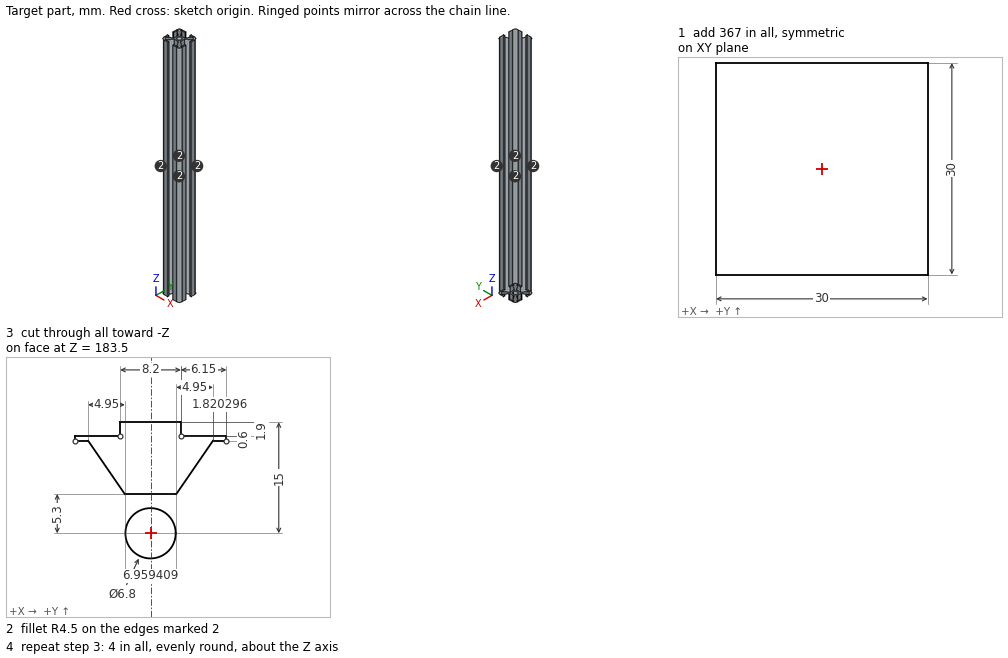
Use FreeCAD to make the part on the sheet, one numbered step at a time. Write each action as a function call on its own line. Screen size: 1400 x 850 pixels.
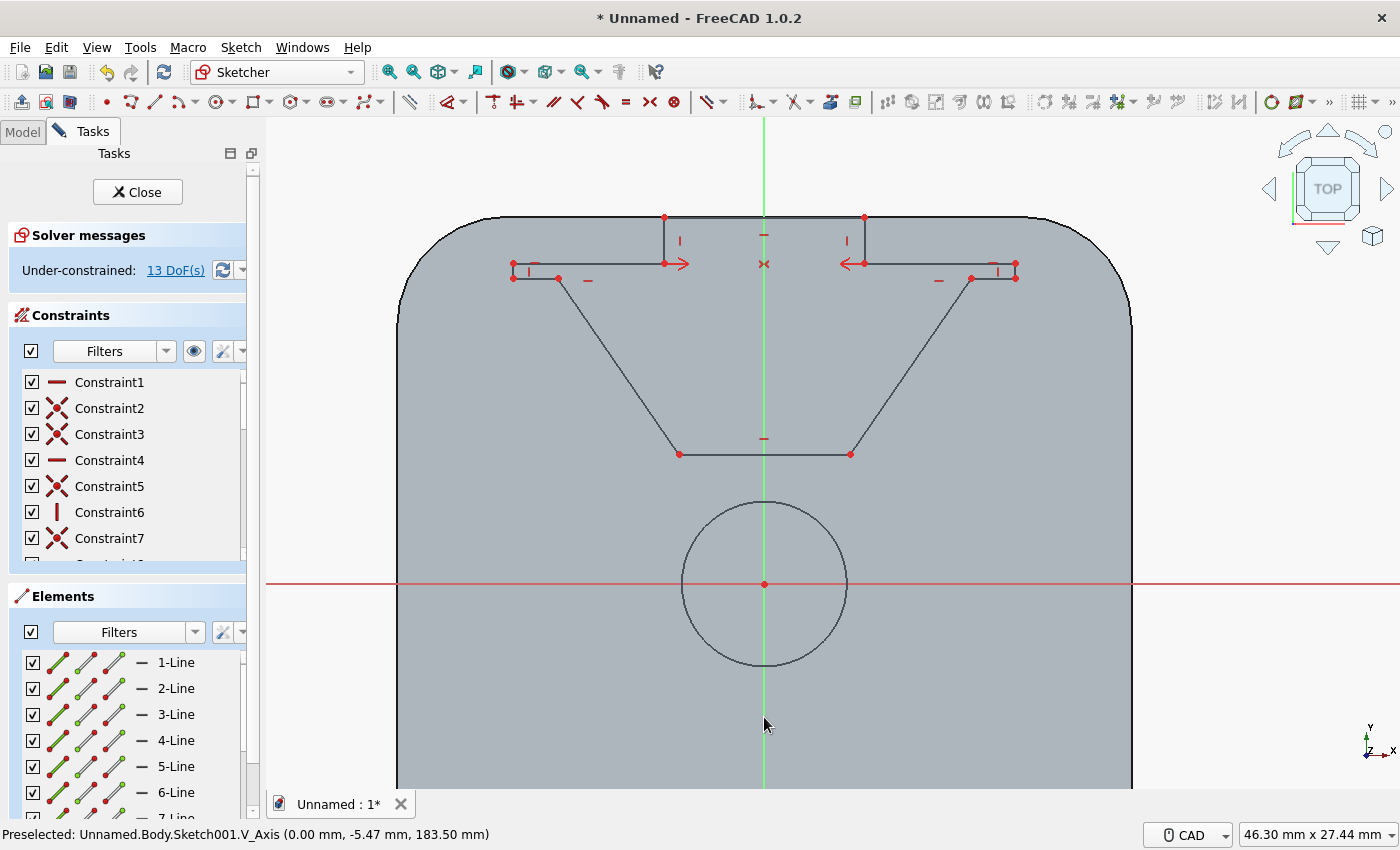
click(1015, 279)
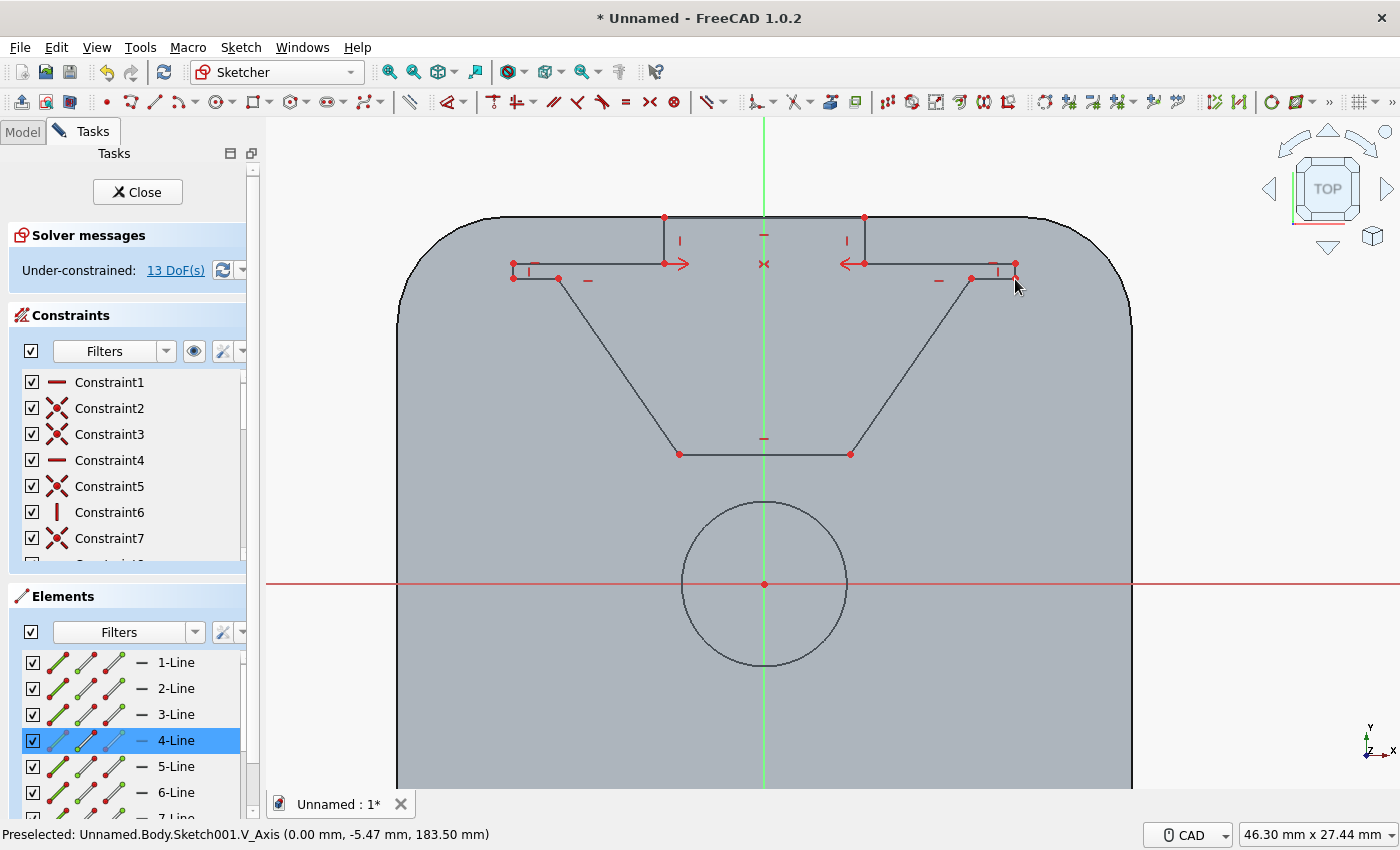
click(513, 279)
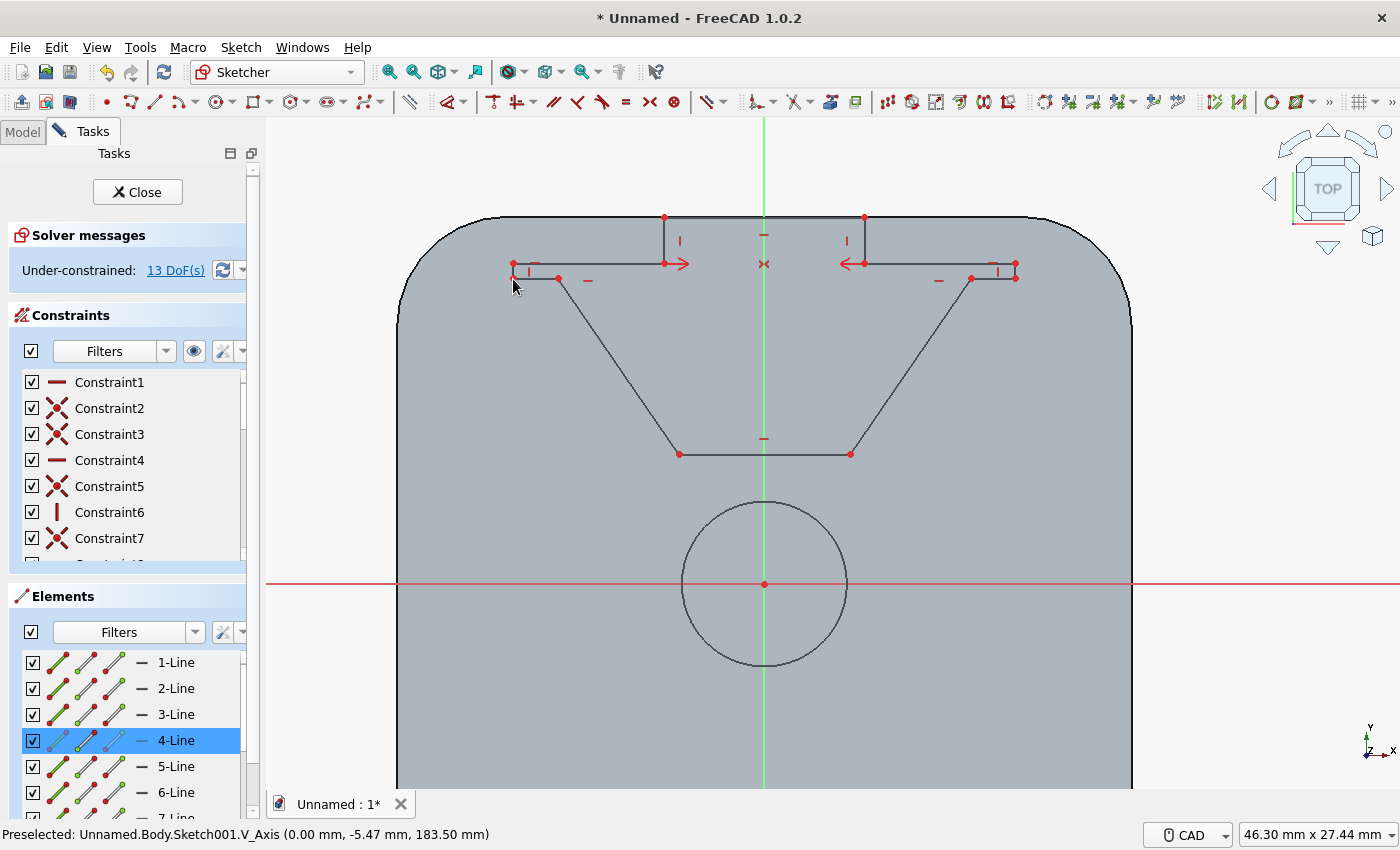
click(764, 717)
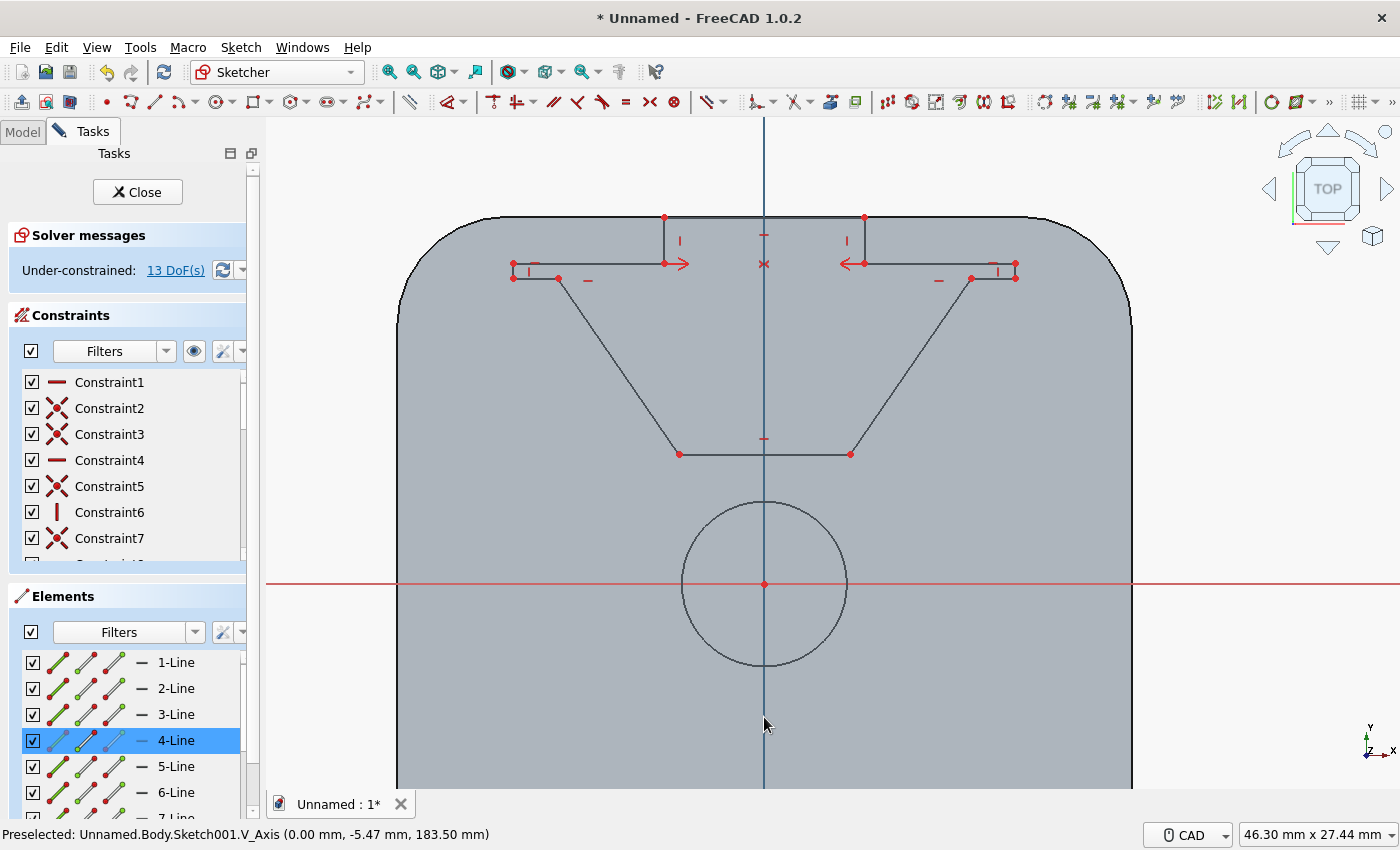
key(s)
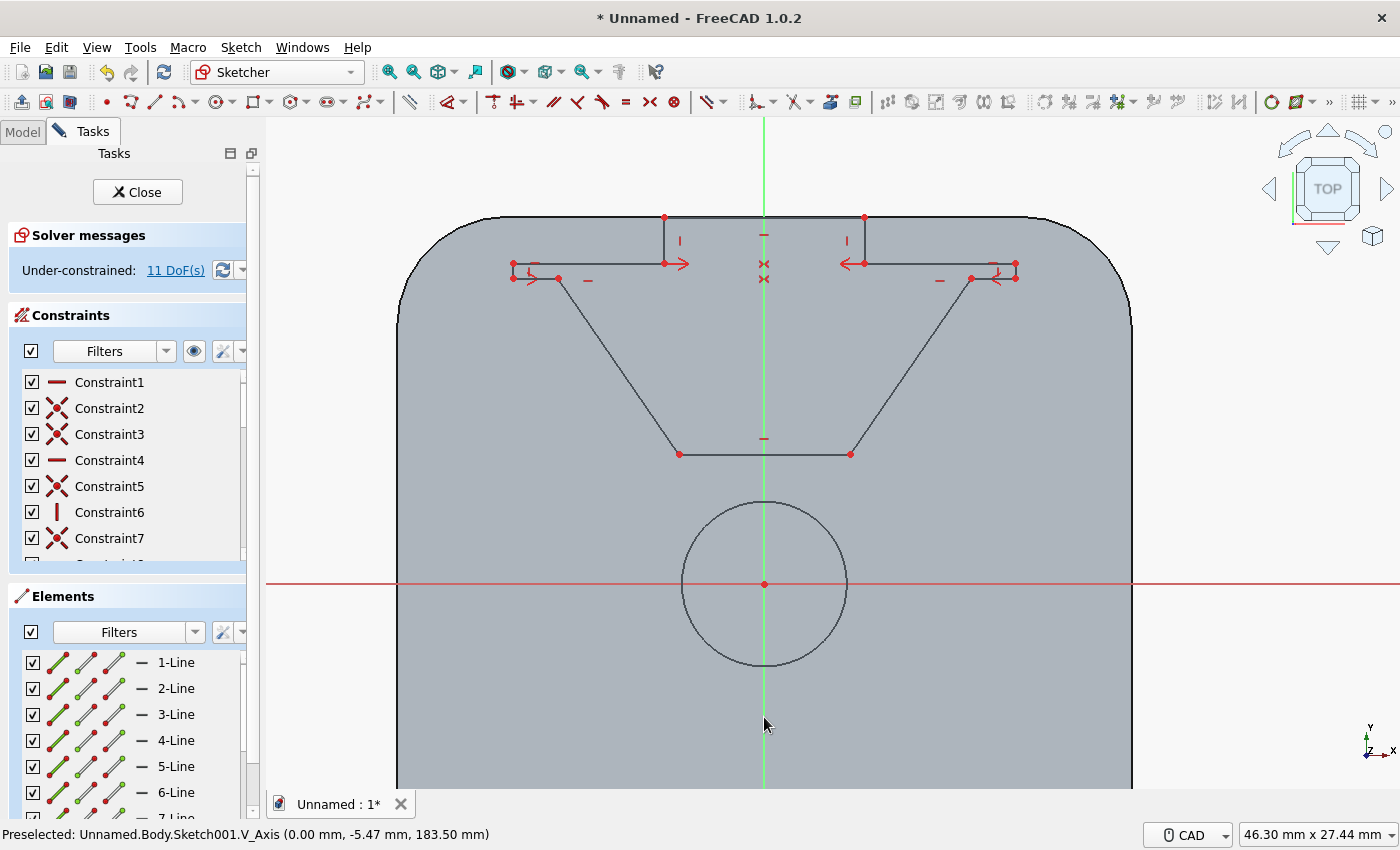
key(d)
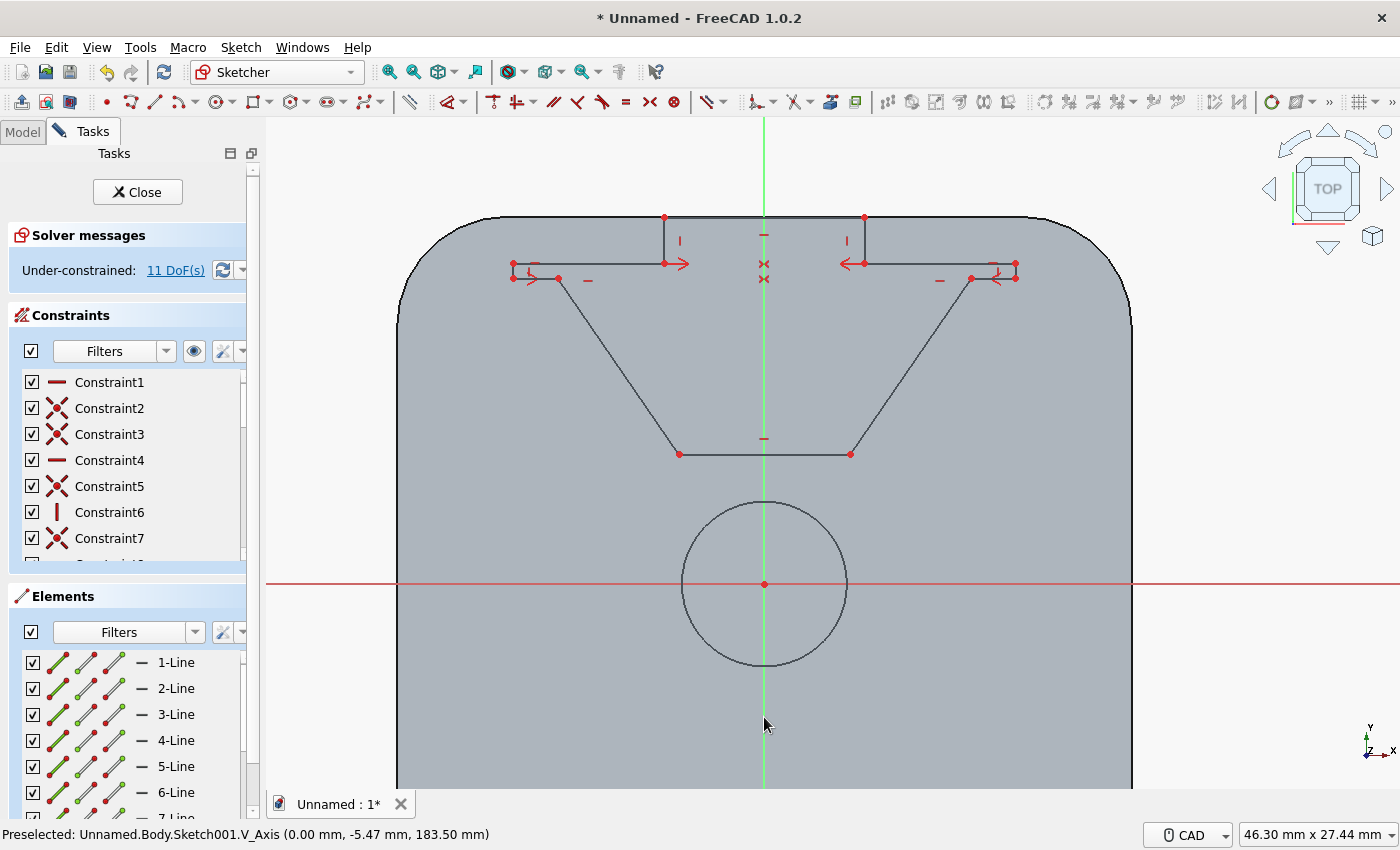
click(823, 526)
click(846, 503)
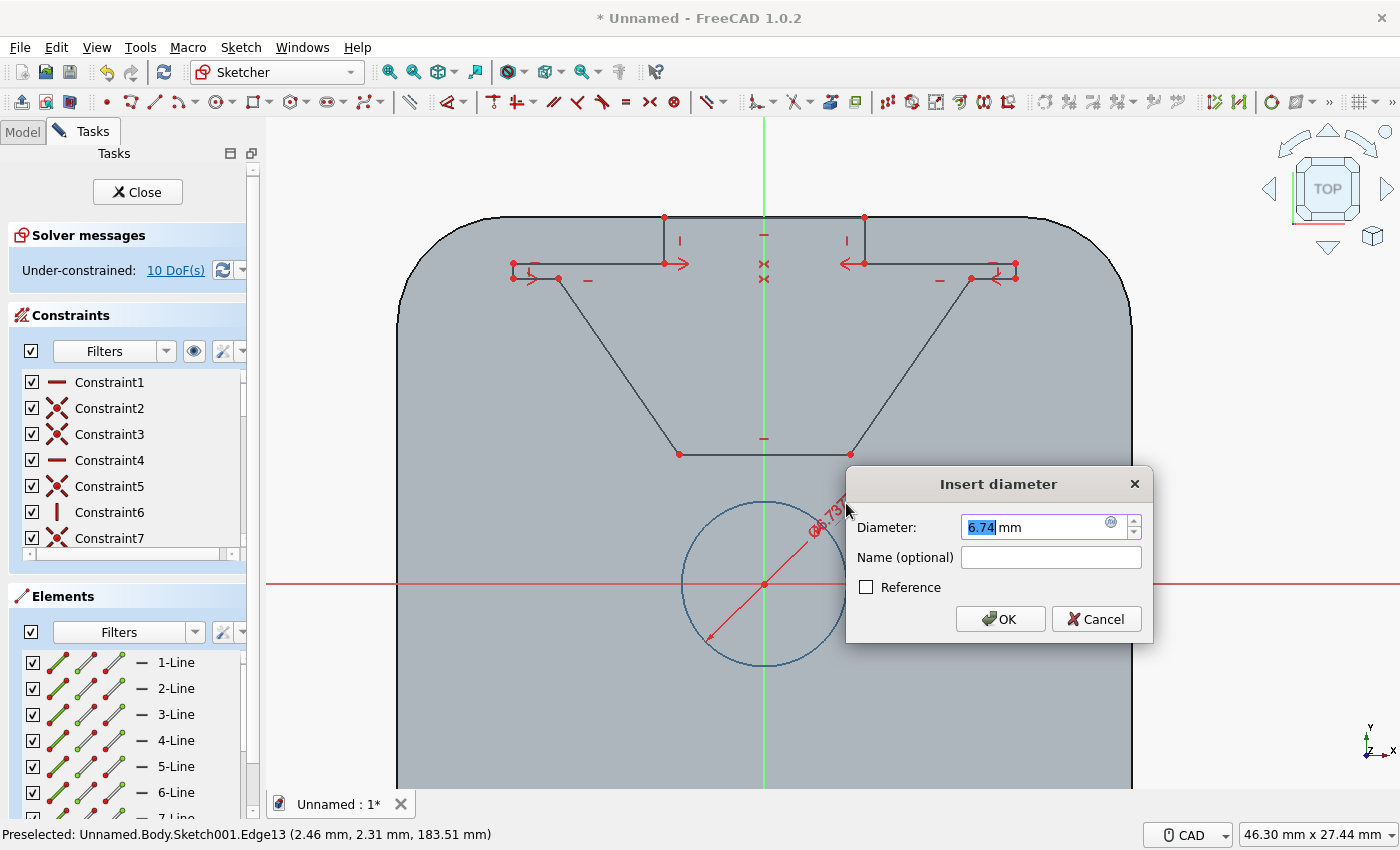
text(6.8)
key(Return)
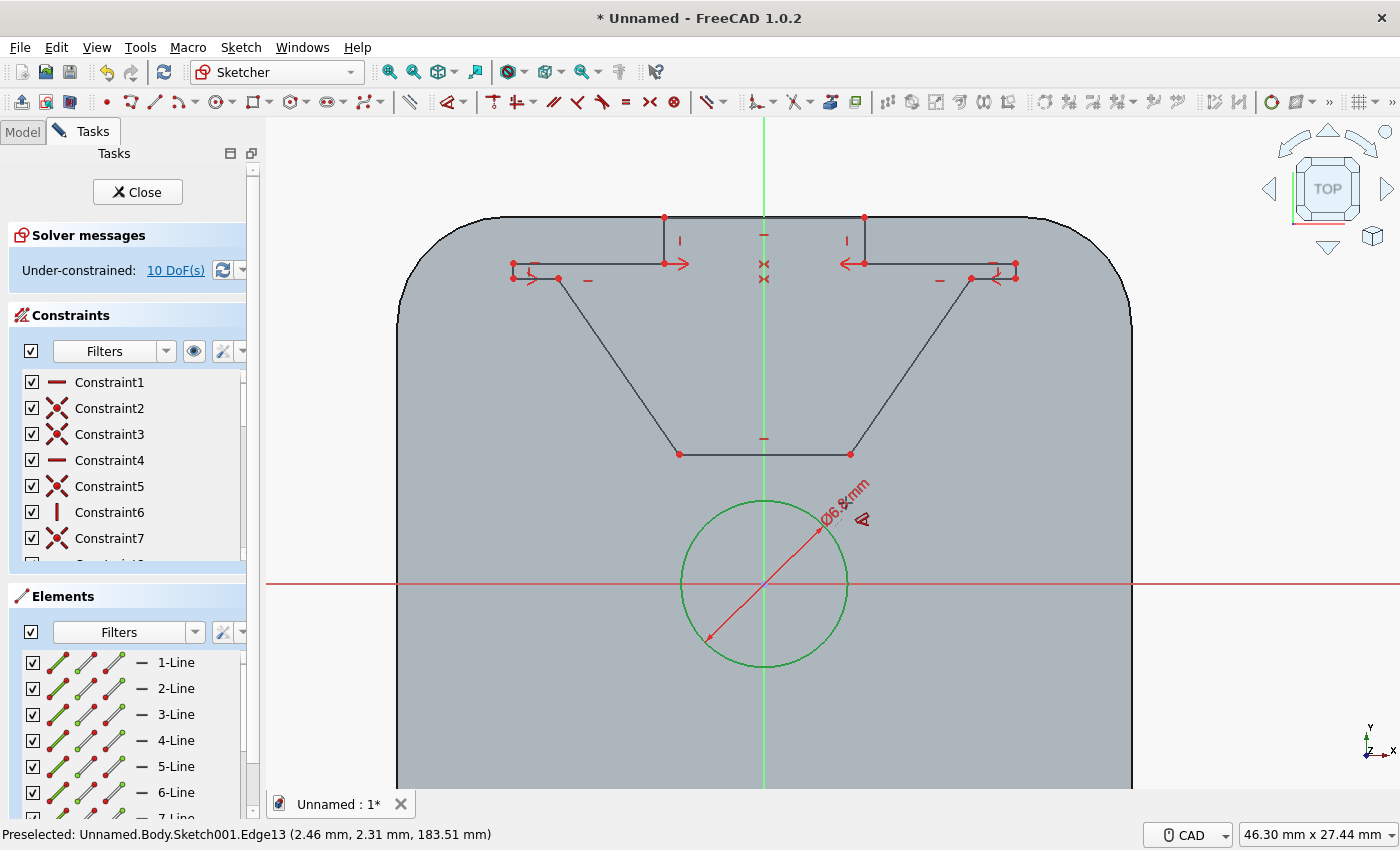
scroll(1016, 271, up, 5)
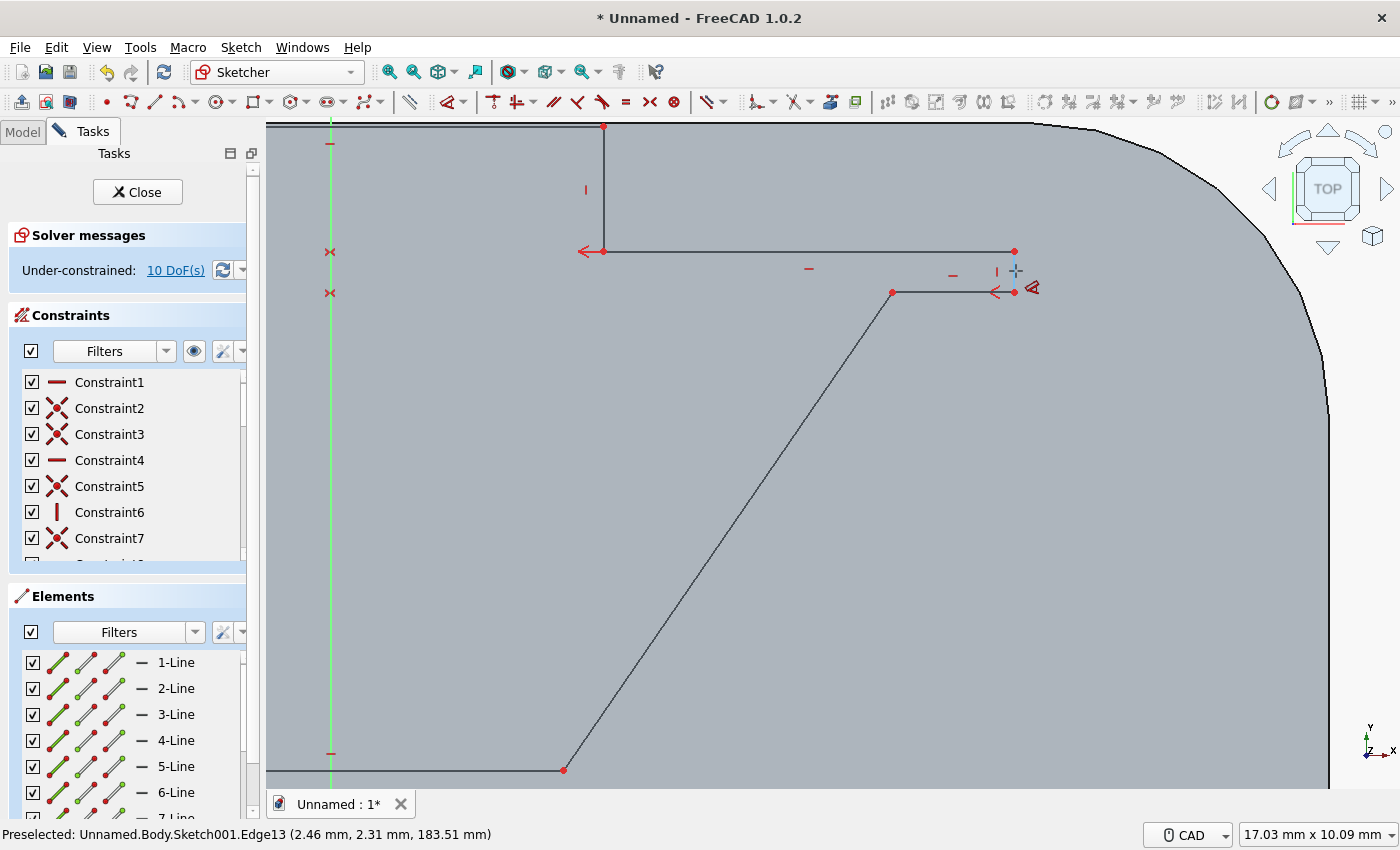
click(1014, 272)
click(1048, 272)